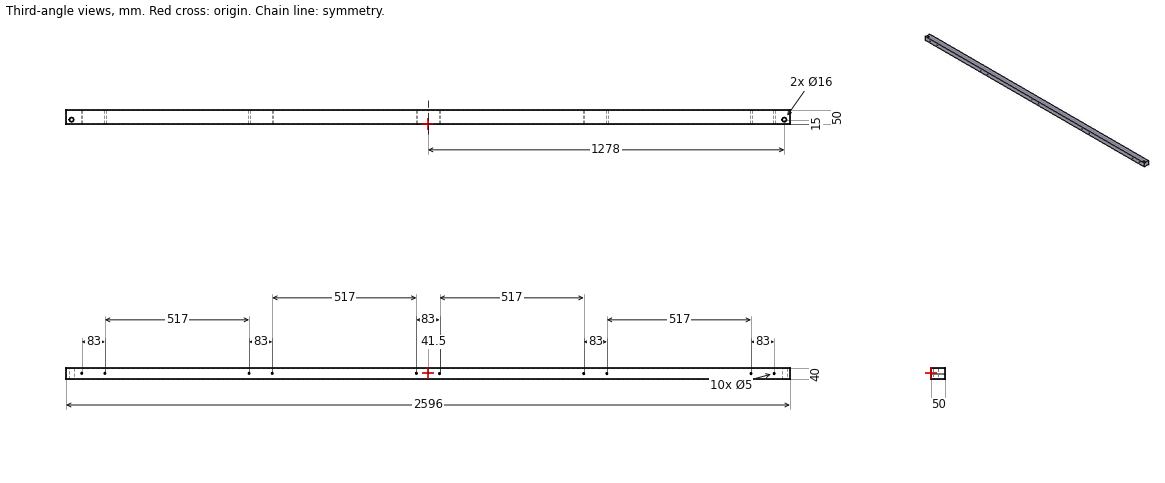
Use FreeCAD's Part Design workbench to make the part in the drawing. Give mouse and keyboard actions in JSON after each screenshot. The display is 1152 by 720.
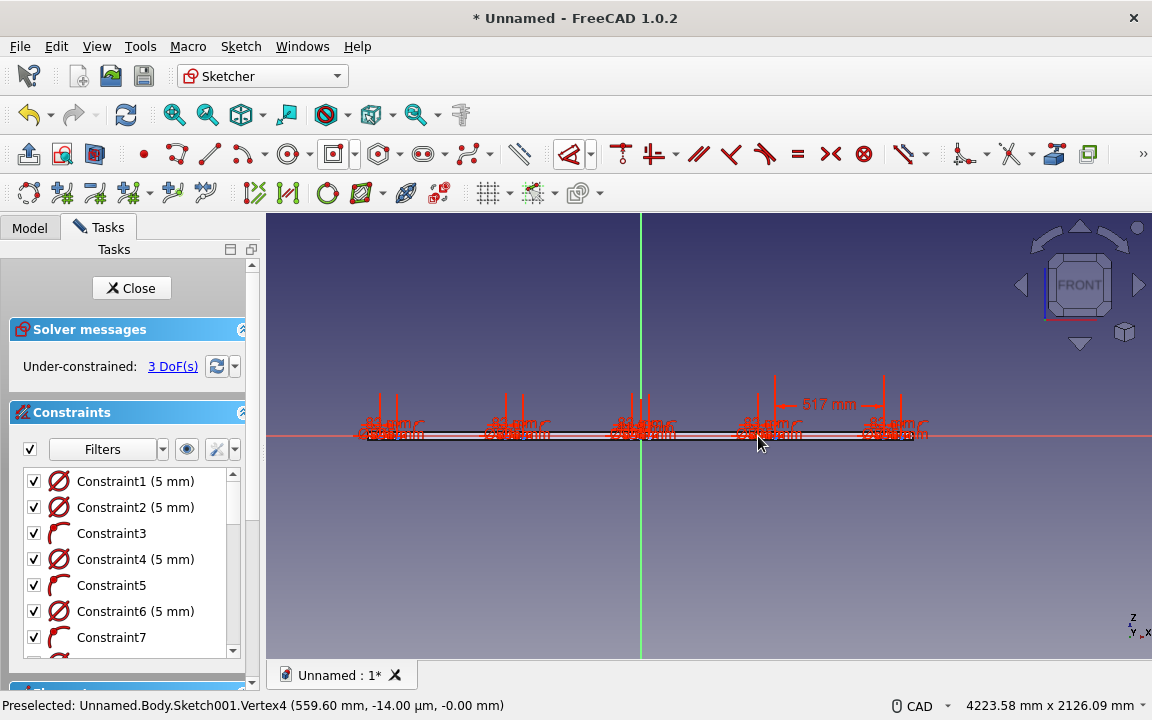
{"action": "scroll", "coordinate": [649, 436], "scroll_direction": "up", "scroll_amount": 2}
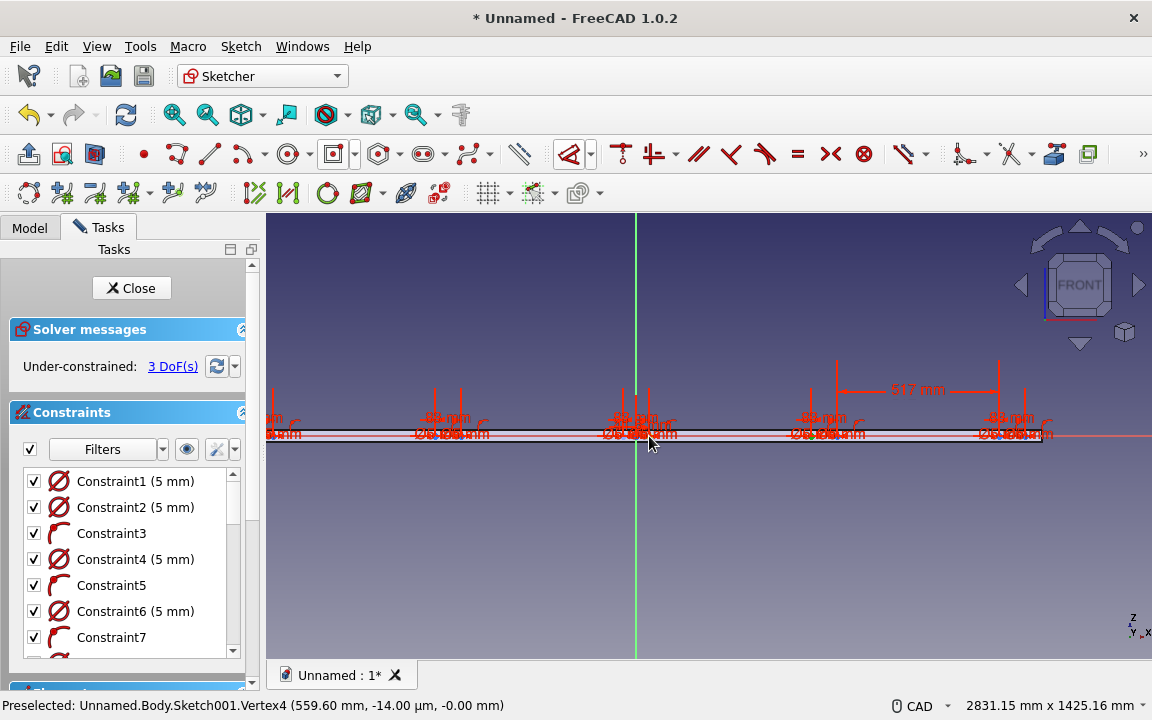
{"action": "left_click", "coordinate": [649, 436]}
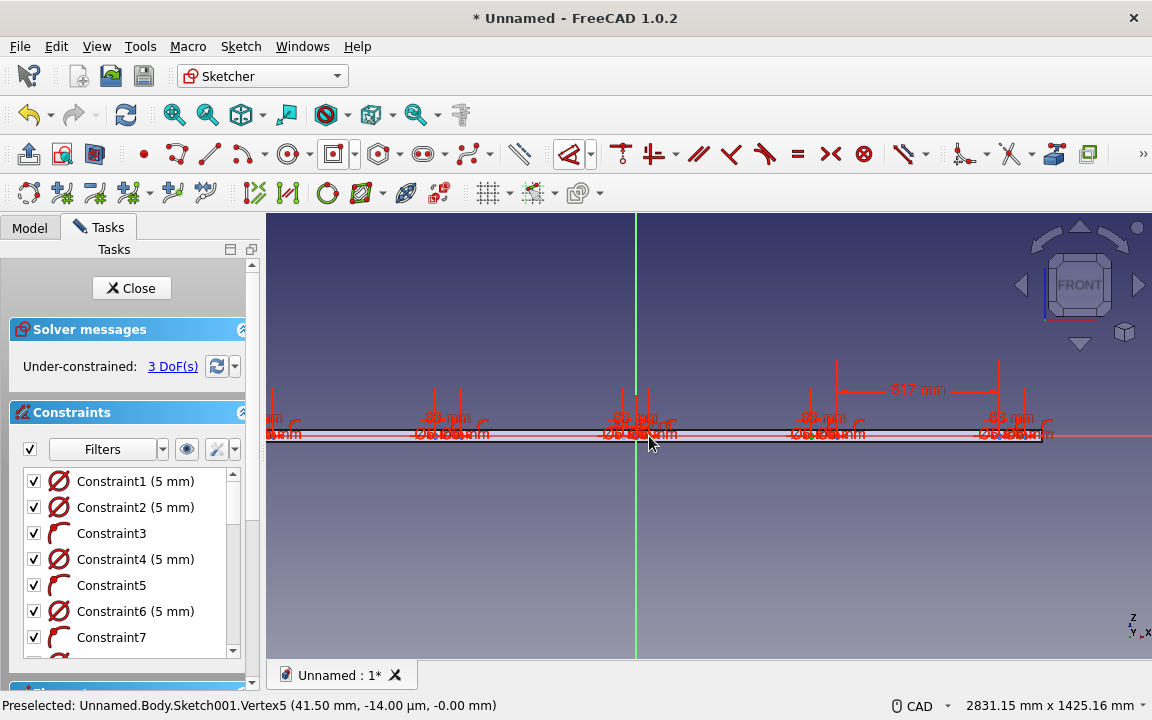
{"action": "left_click", "coordinate": [590, 154]}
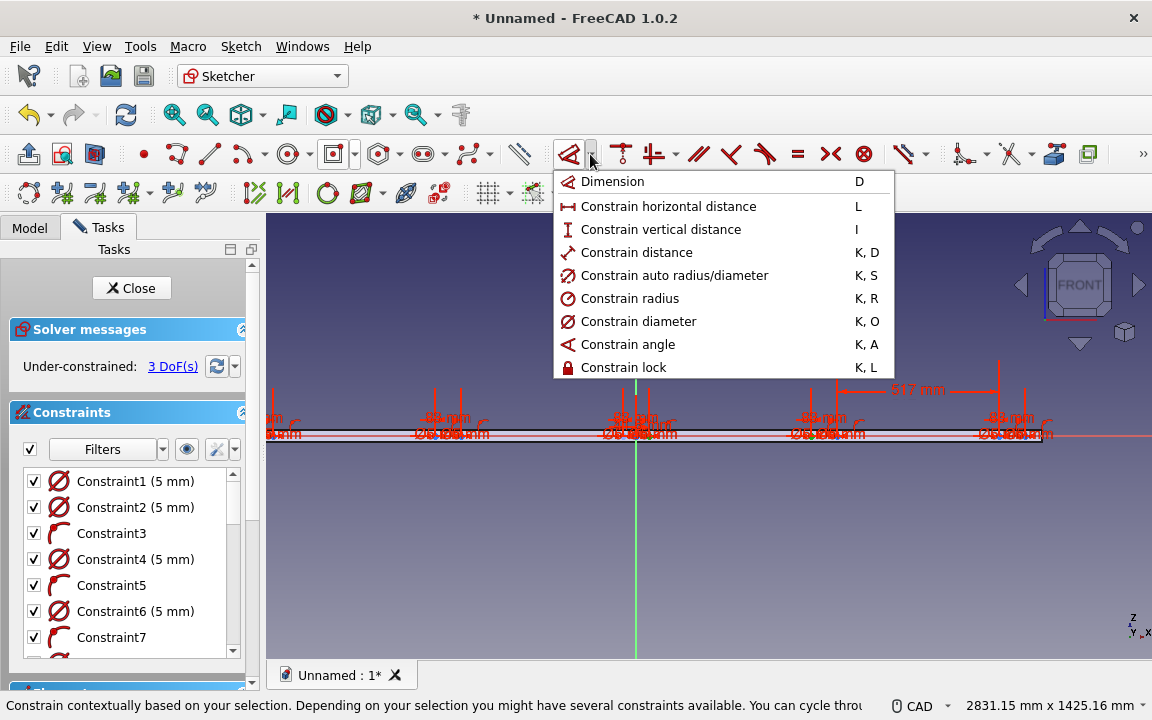
{"action": "left_click", "coordinate": [724, 206]}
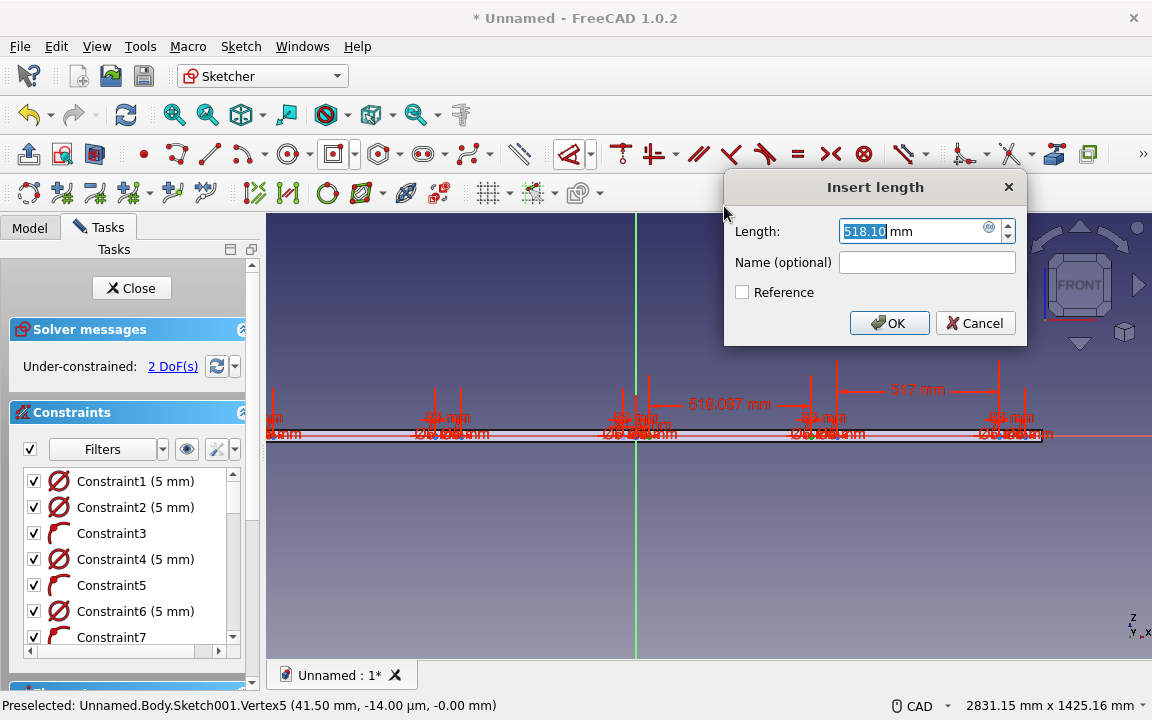
{"action": "type", "text": "517"}
{"action": "key", "text": "Return"}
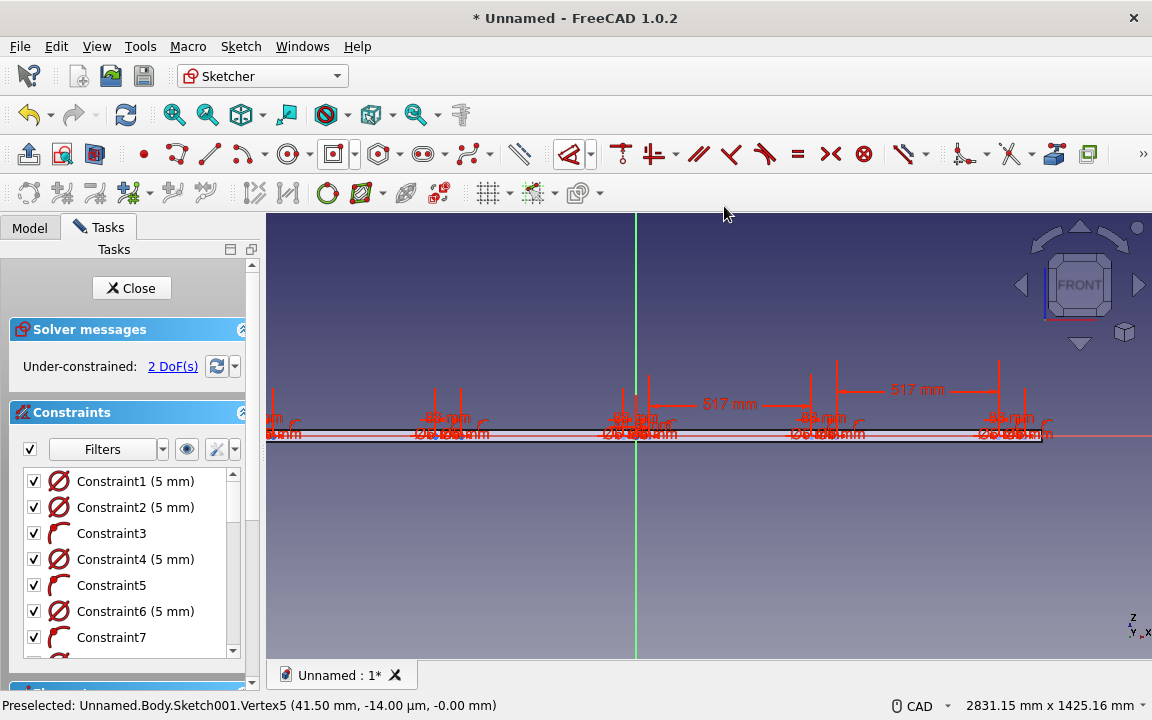
{"action": "left_click", "coordinate": [623, 436]}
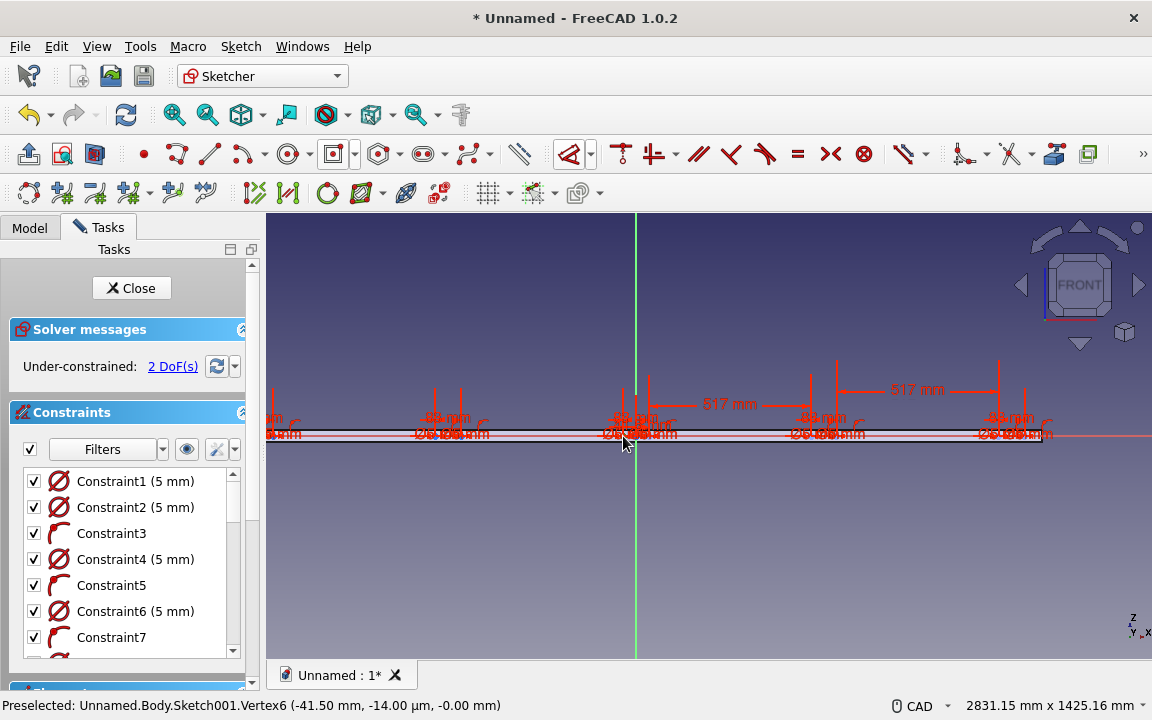
{"action": "left_click", "coordinate": [461, 436]}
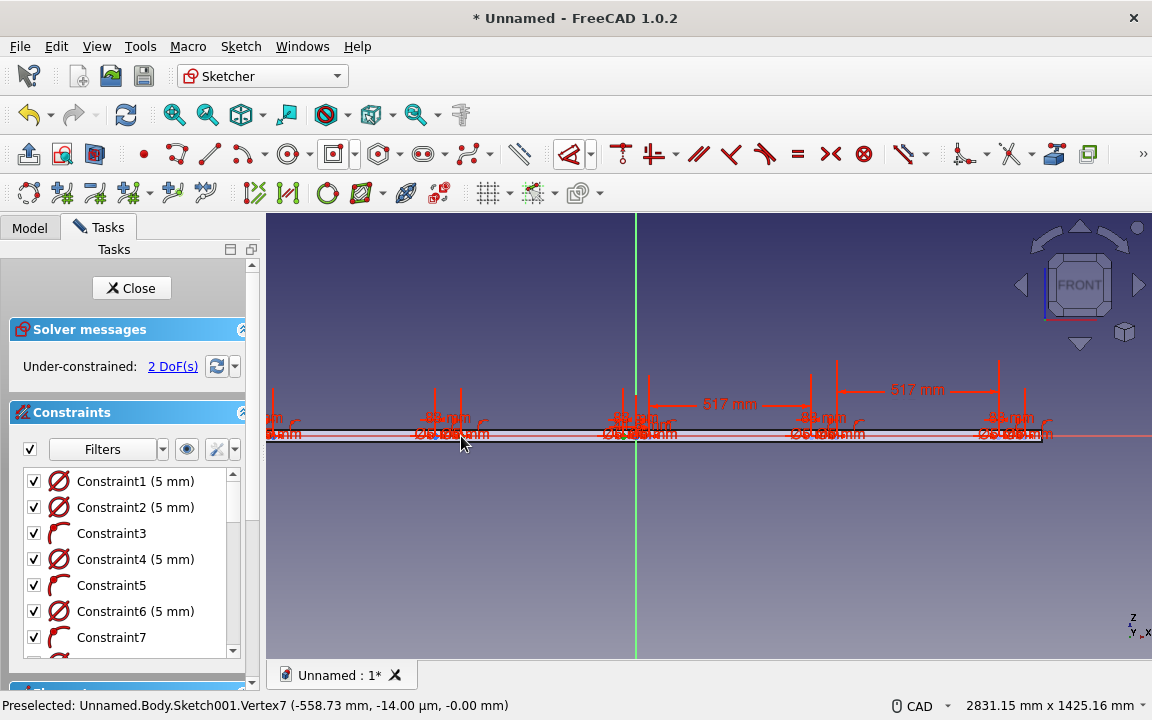
{"action": "left_click", "coordinate": [590, 154]}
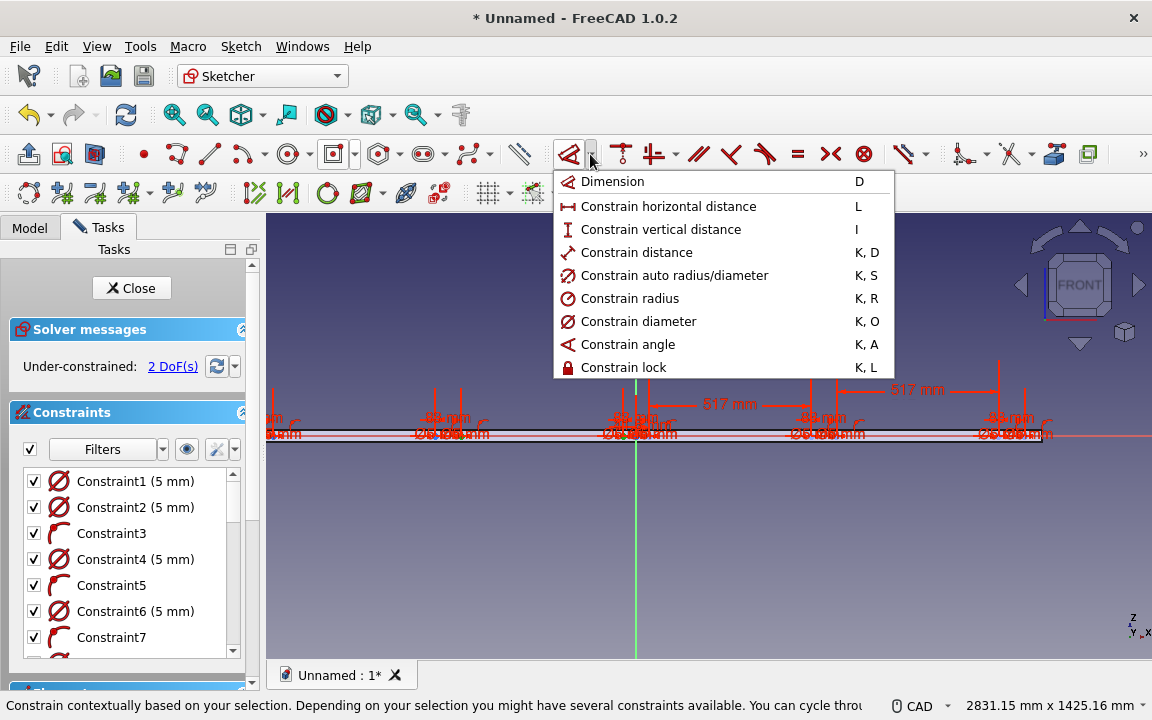
{"action": "left_click", "coordinate": [724, 206]}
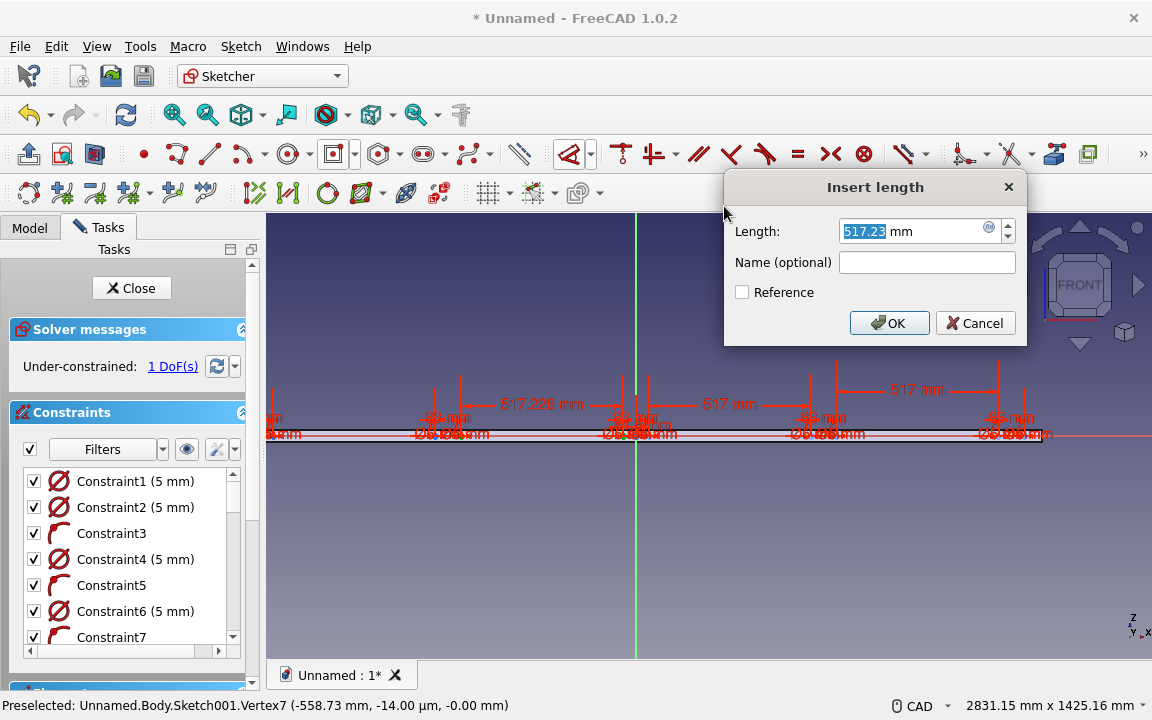
{"action": "type", "text": "517"}
{"action": "key", "text": "Return"}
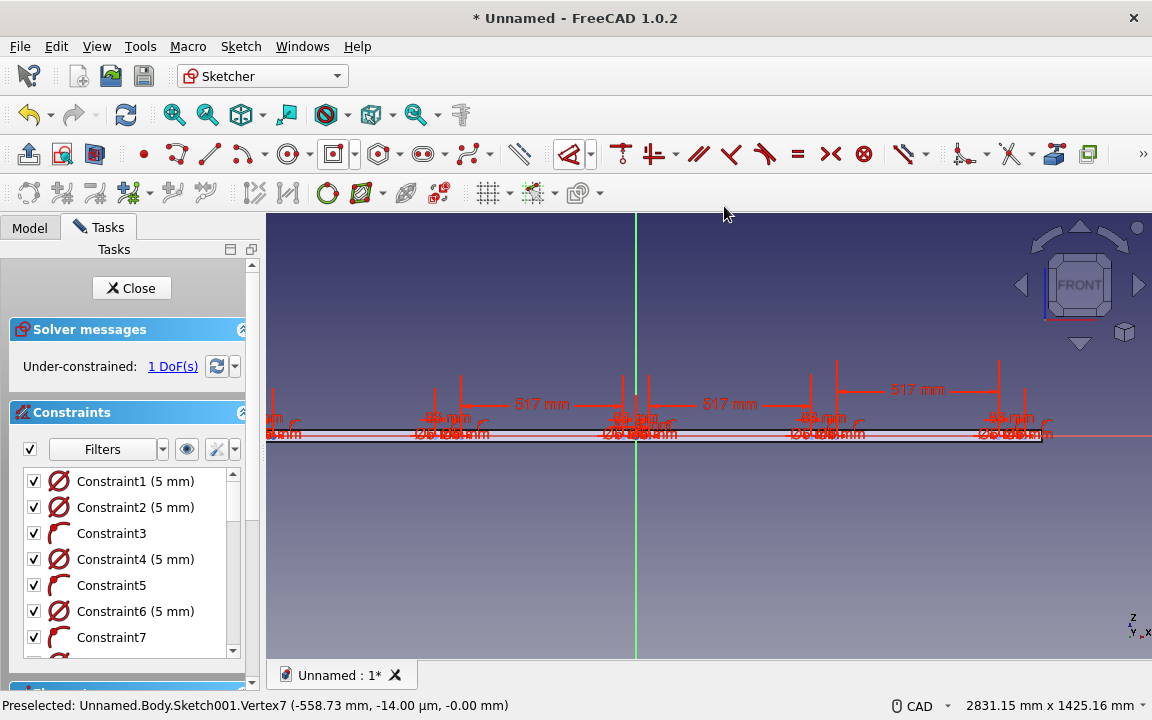
{"action": "left_click", "coordinate": [435, 436]}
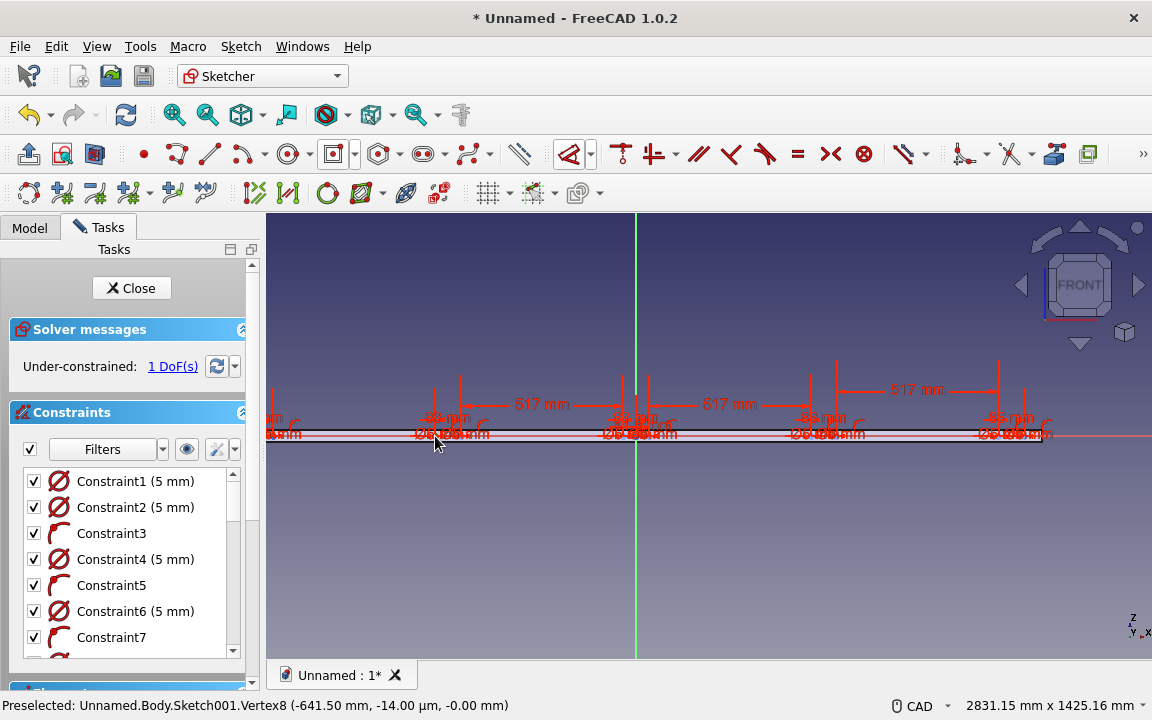
{"action": "scroll", "coordinate": [649, 436], "scroll_direction": "down", "scroll_amount": 2}